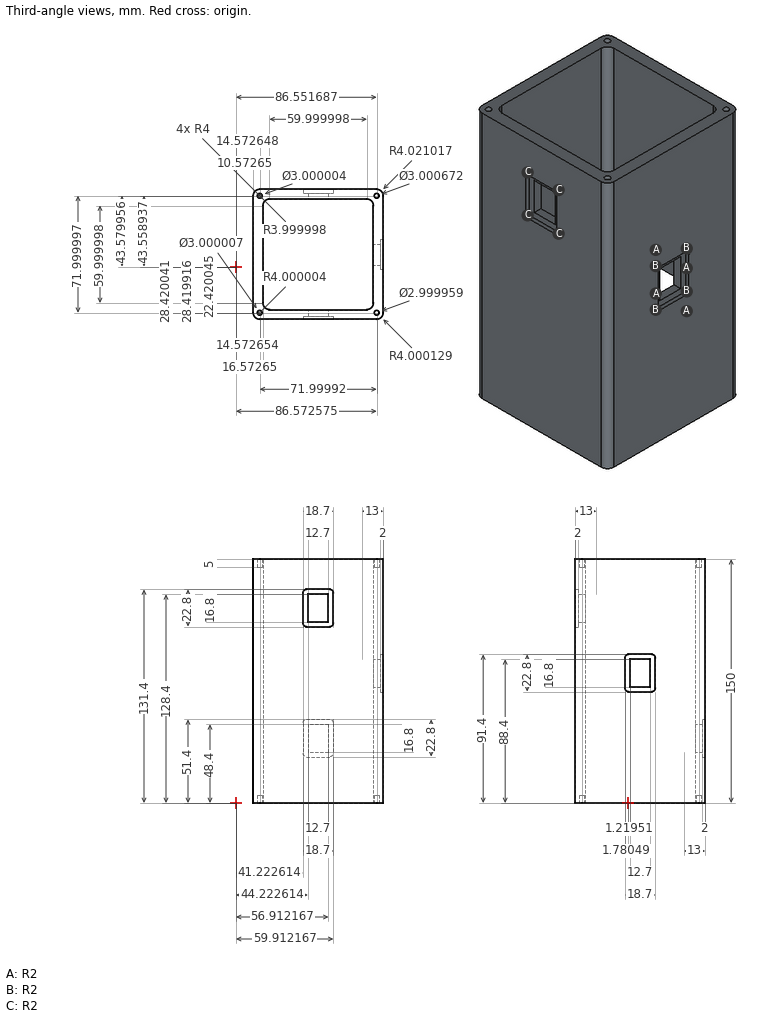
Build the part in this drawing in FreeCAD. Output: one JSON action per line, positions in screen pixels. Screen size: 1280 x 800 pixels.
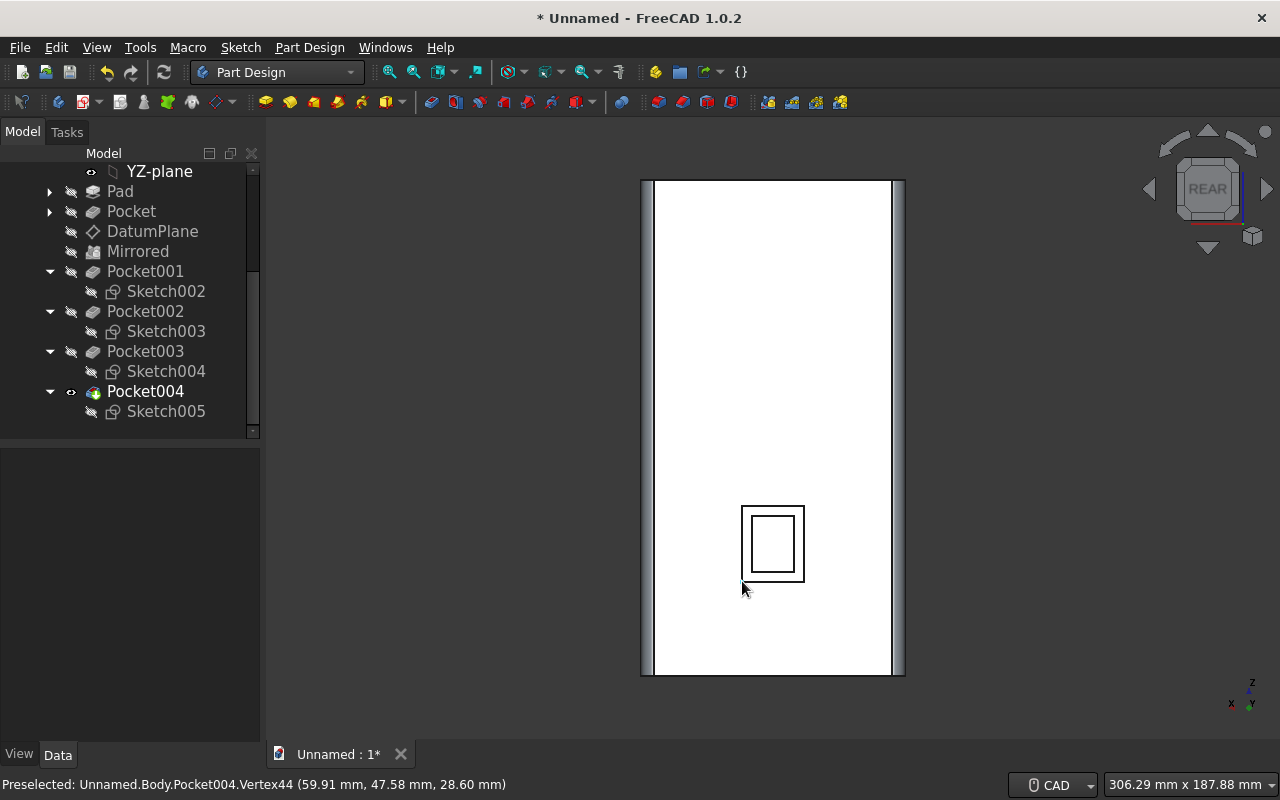
{"action": "key", "text": "6"}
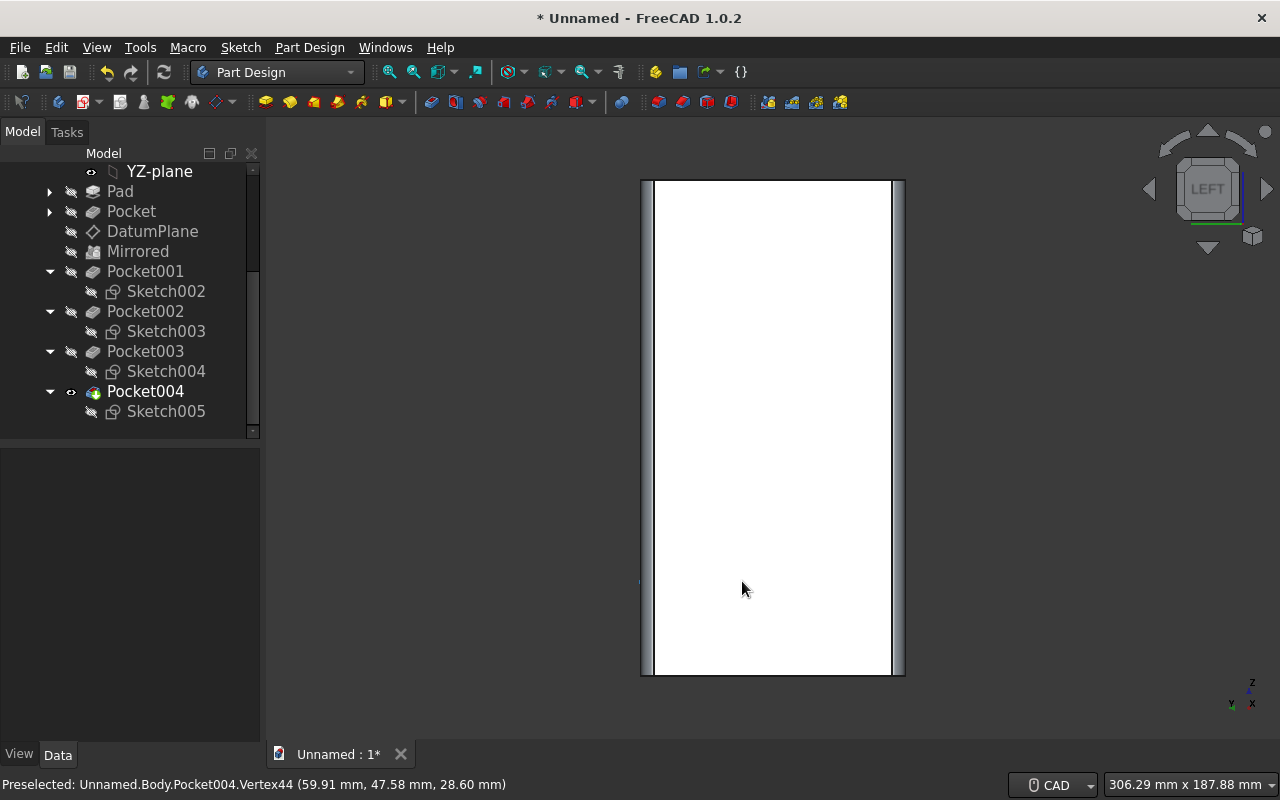
{"action": "scroll", "coordinate": [644, 581], "scroll_direction": "up", "scroll_amount": 9}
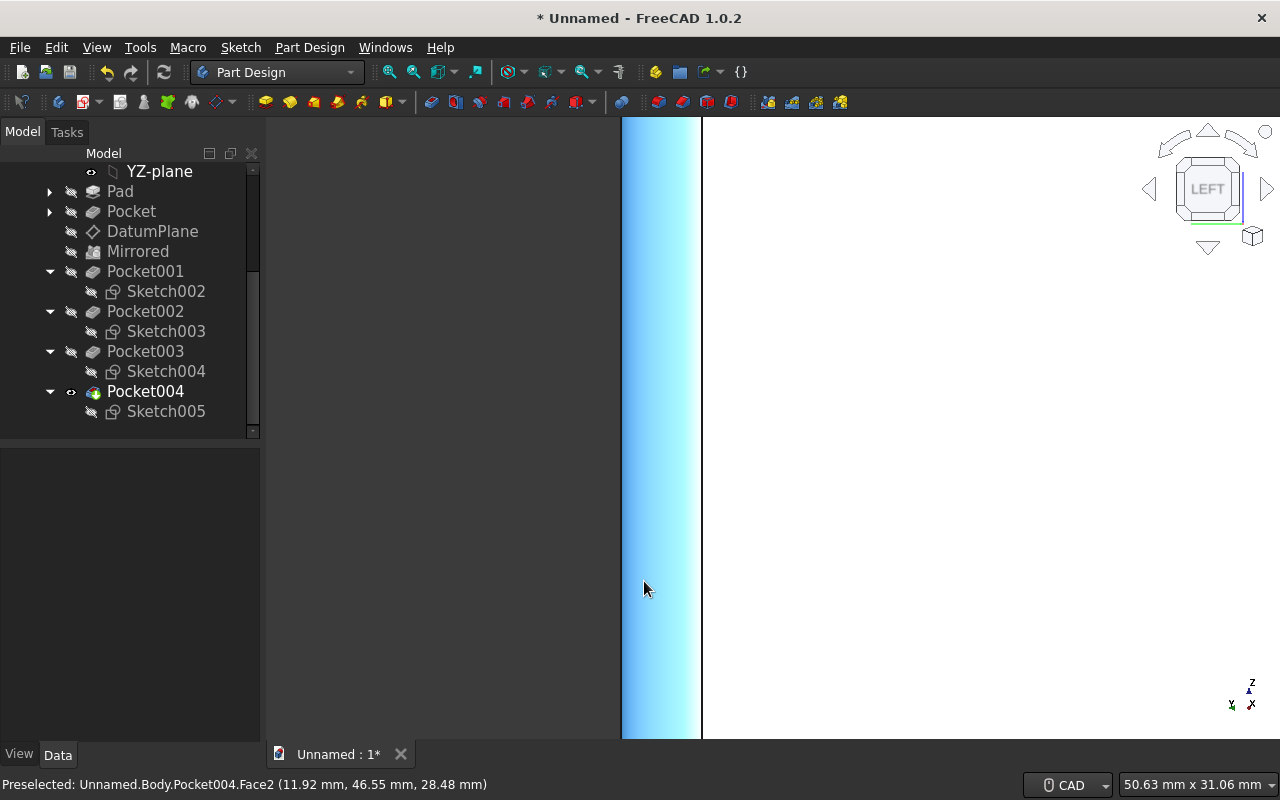
{"action": "key", "text": "v f"}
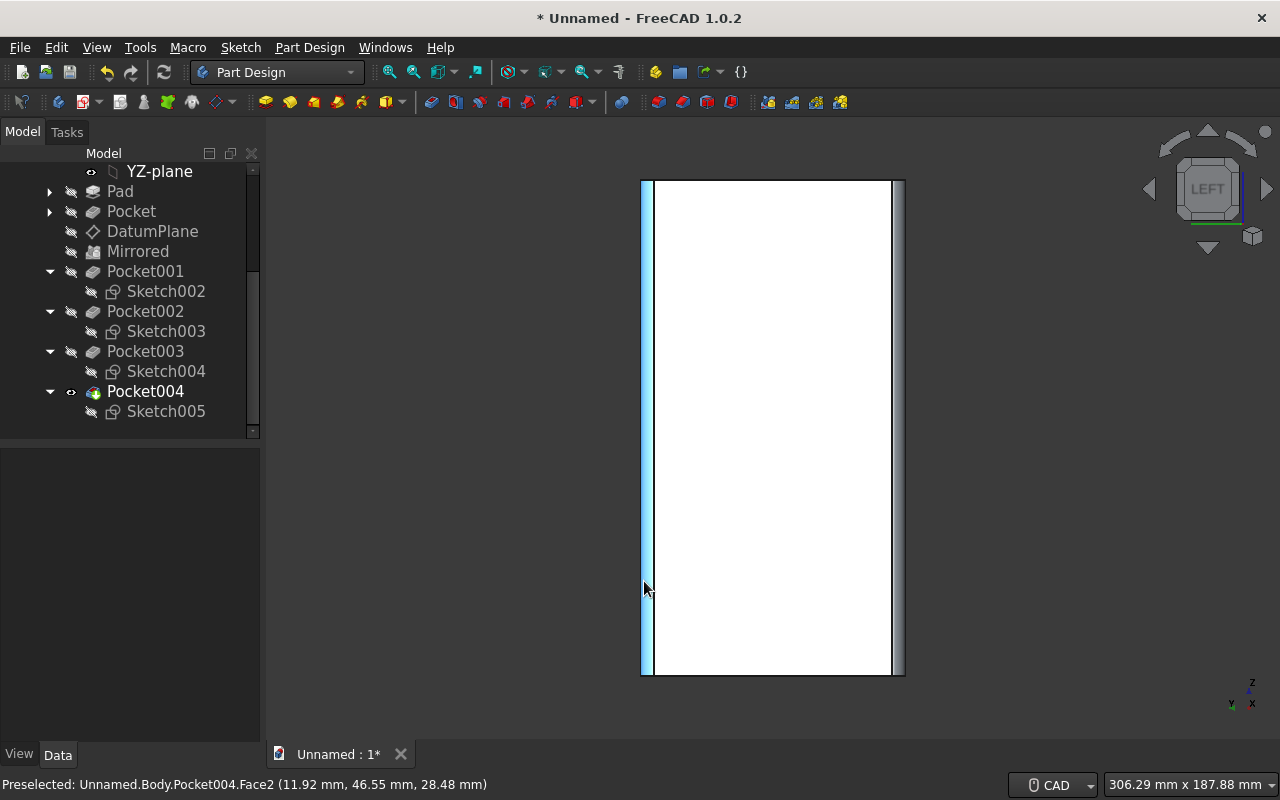
{"action": "key", "text": "v 3"}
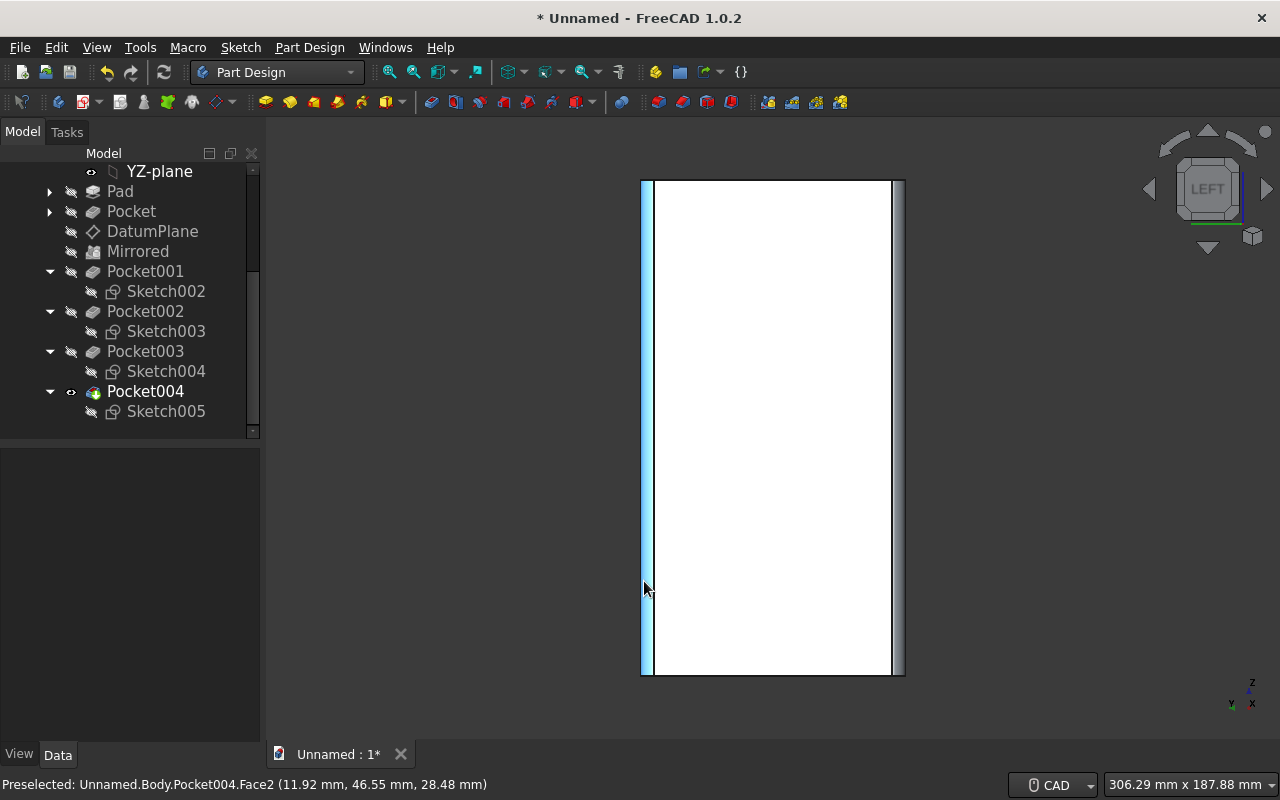
{"action": "key", "text": "0"}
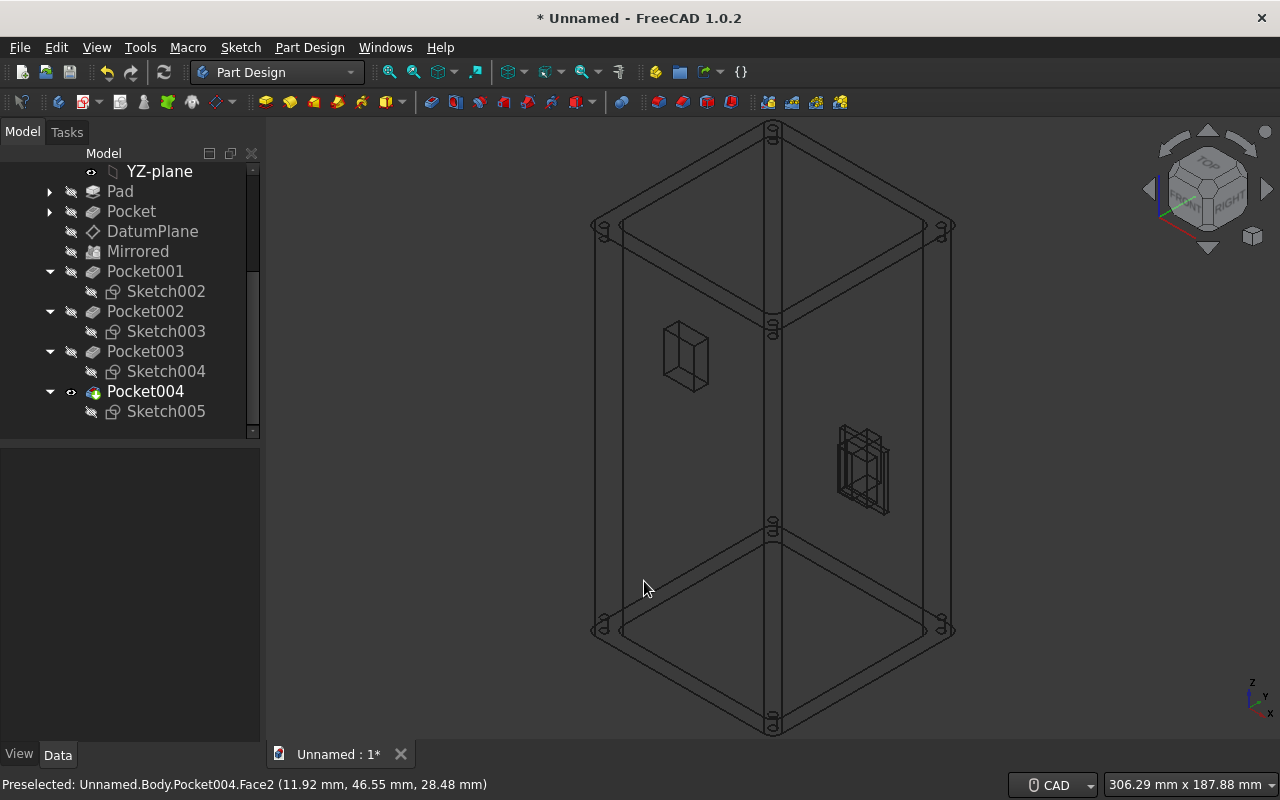
{"action": "key", "text": "v f"}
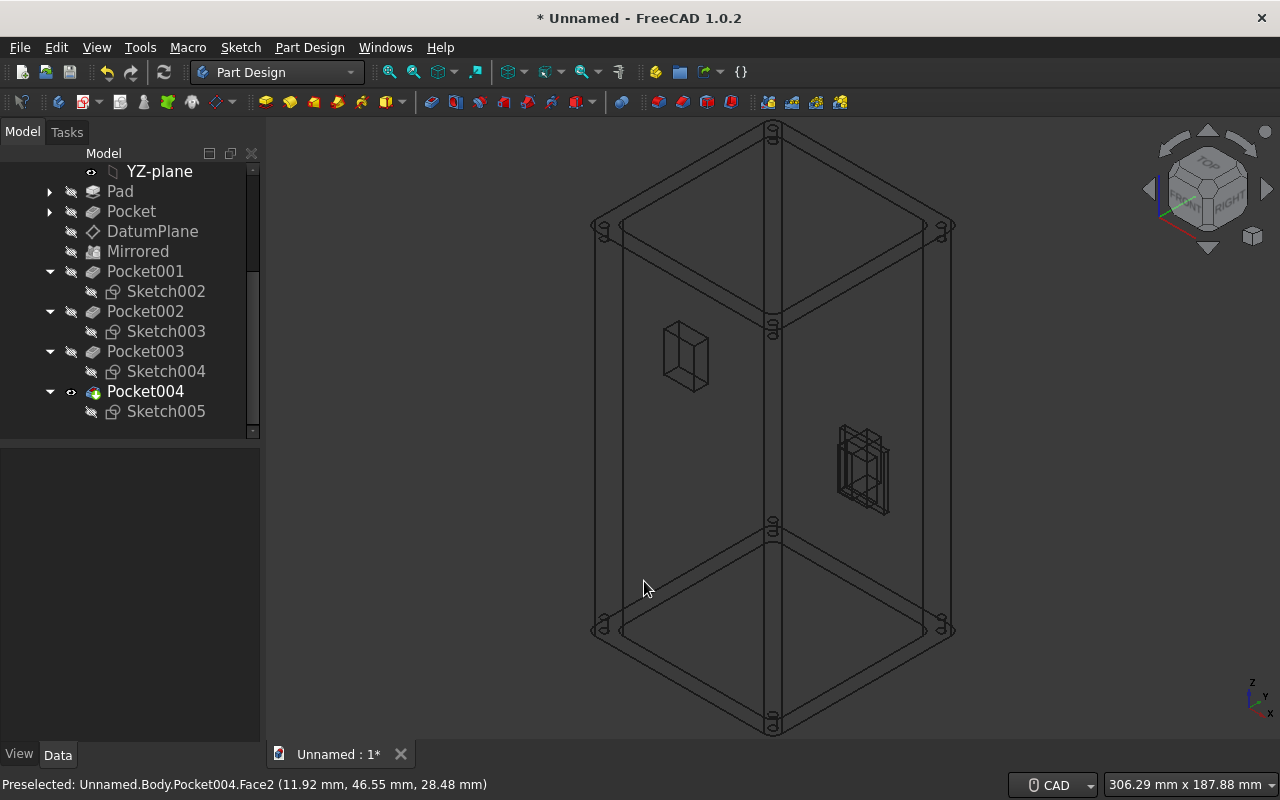
{"action": "scroll", "coordinate": [886, 512], "scroll_direction": "up", "scroll_amount": 9}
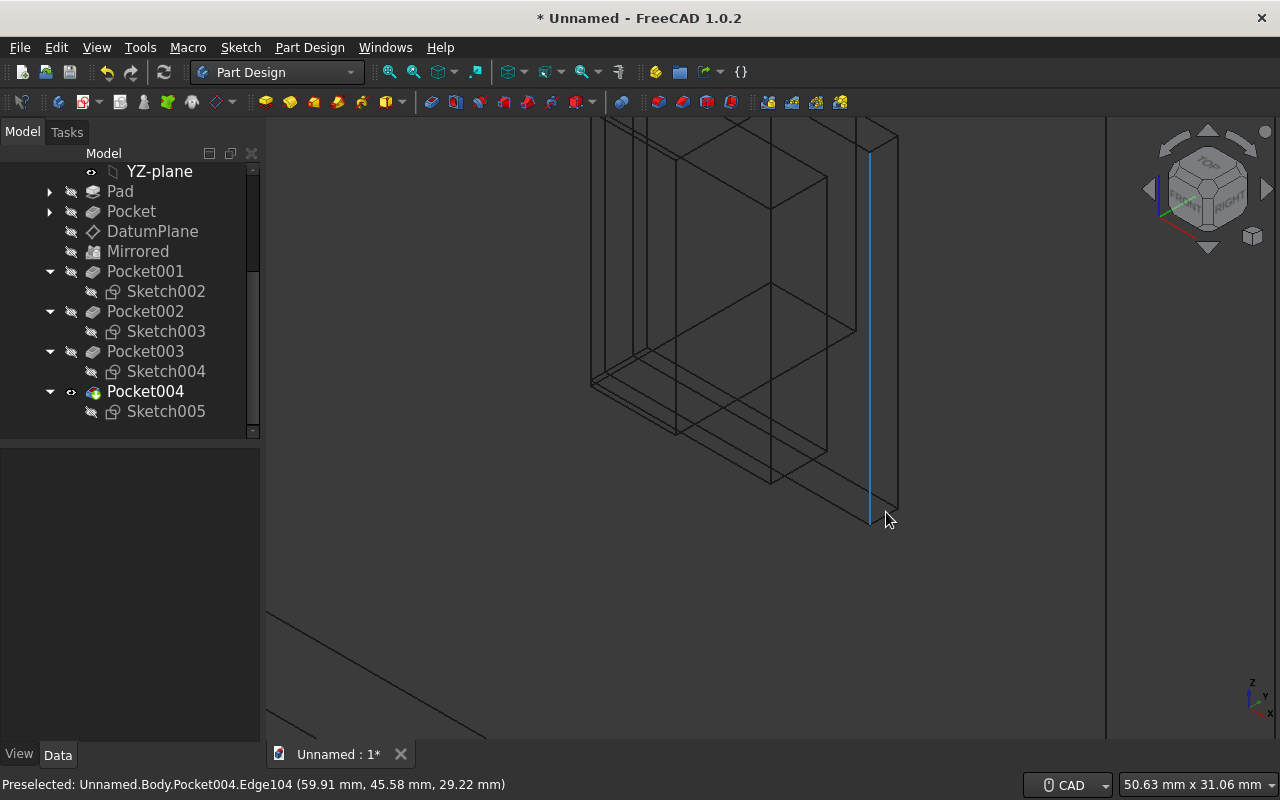
{"action": "left_click", "coordinate": [884, 516]}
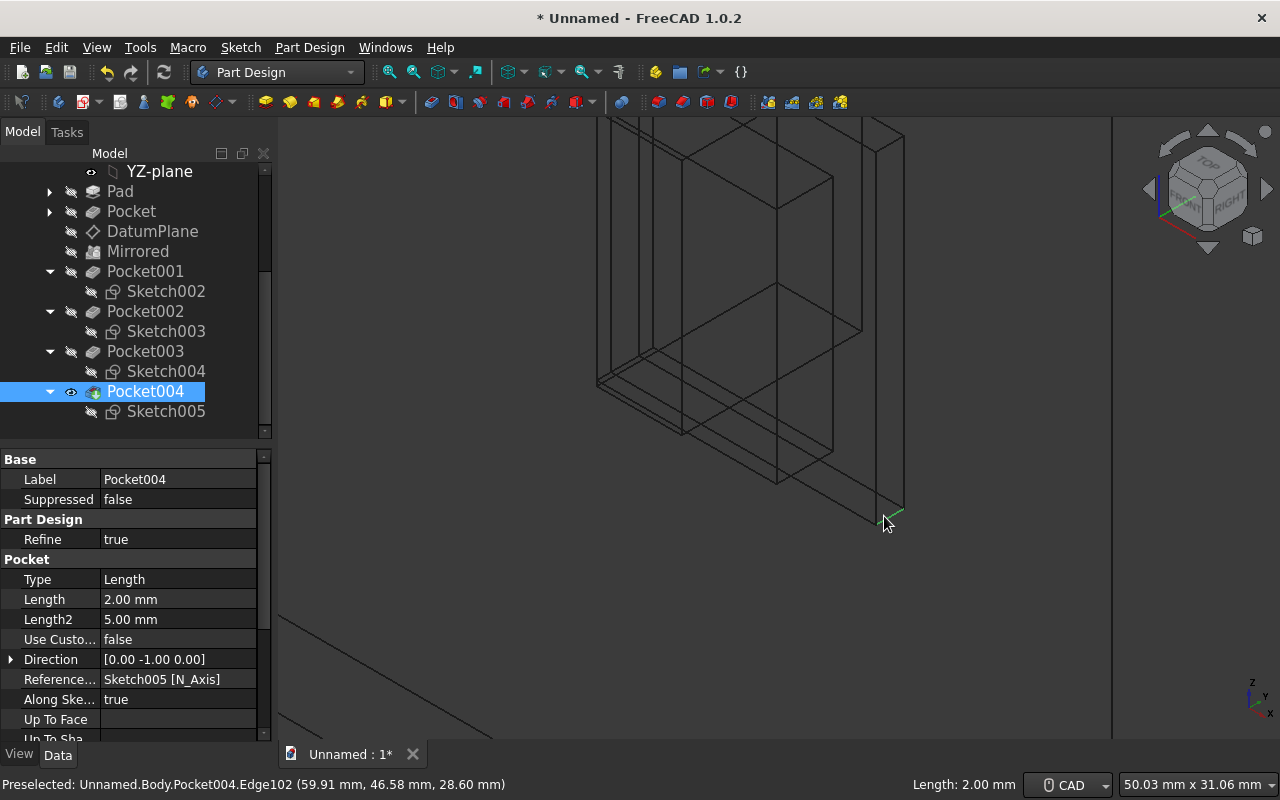
{"action": "left_click", "coordinate": [884, 146], "text": "ctrl"}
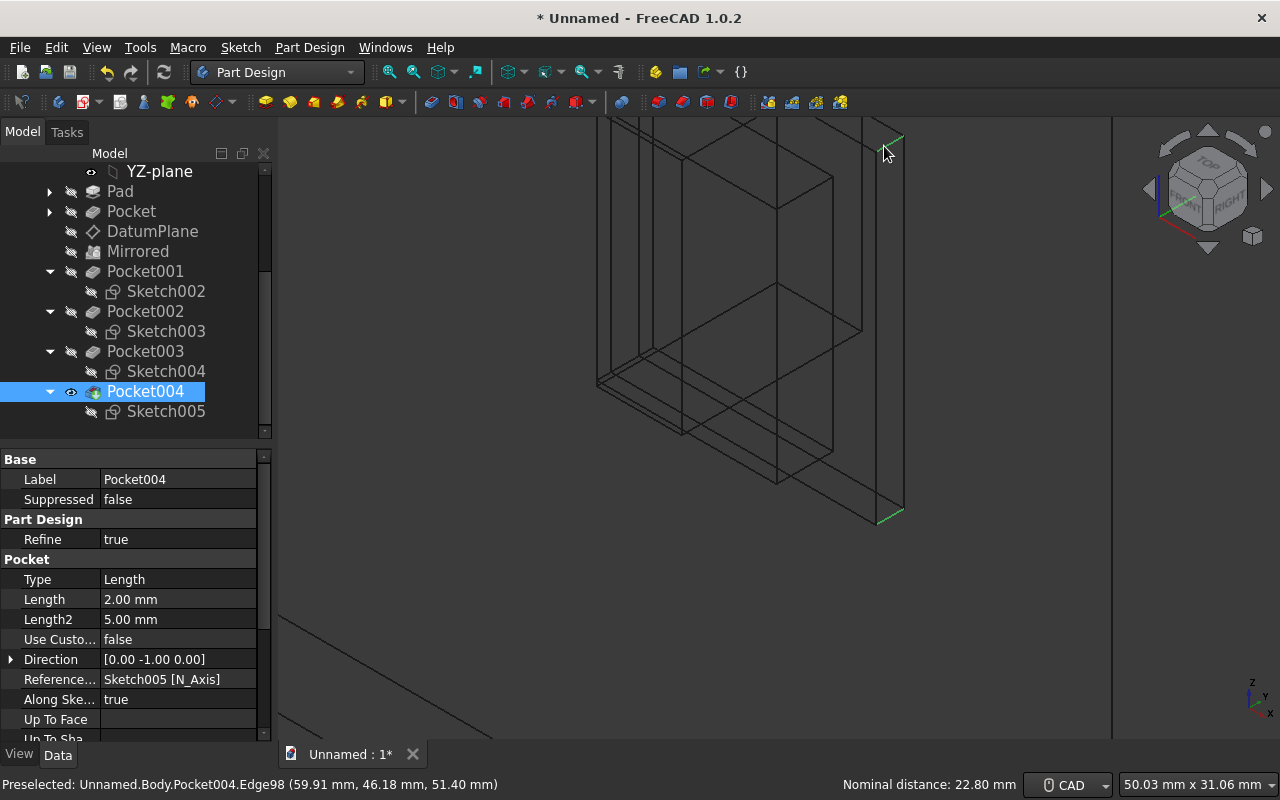
{"action": "left_click", "coordinate": [390, 72]}